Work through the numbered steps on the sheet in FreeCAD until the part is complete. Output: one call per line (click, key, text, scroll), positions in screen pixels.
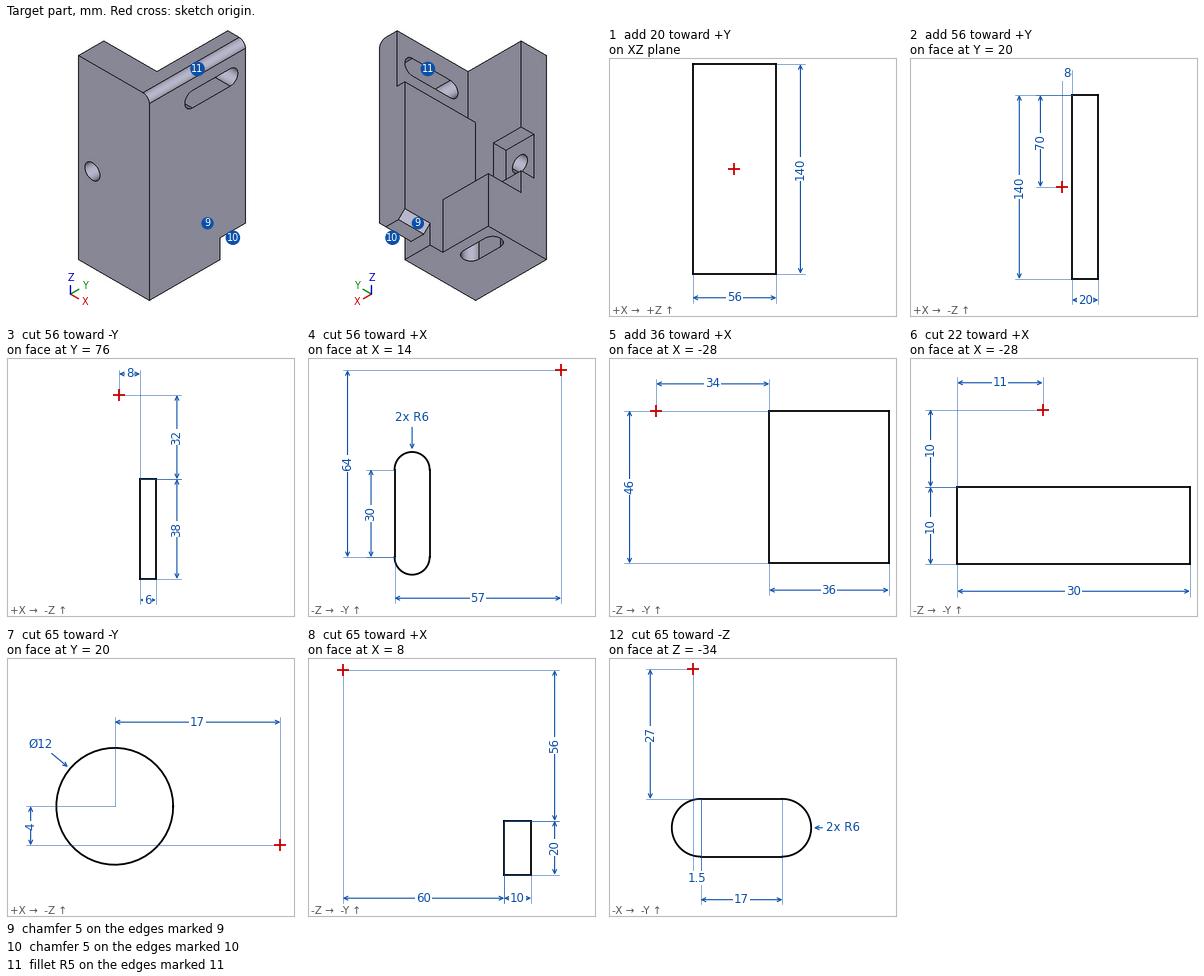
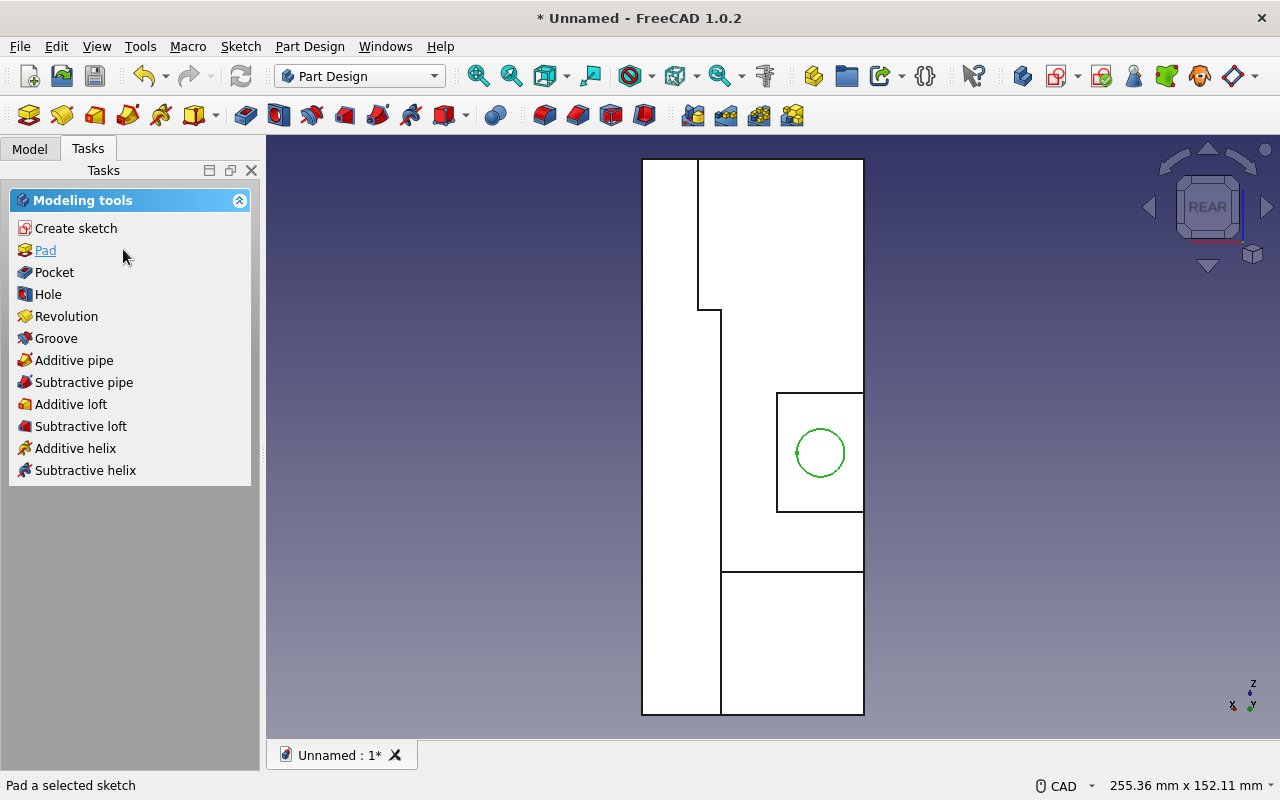
click(246, 116)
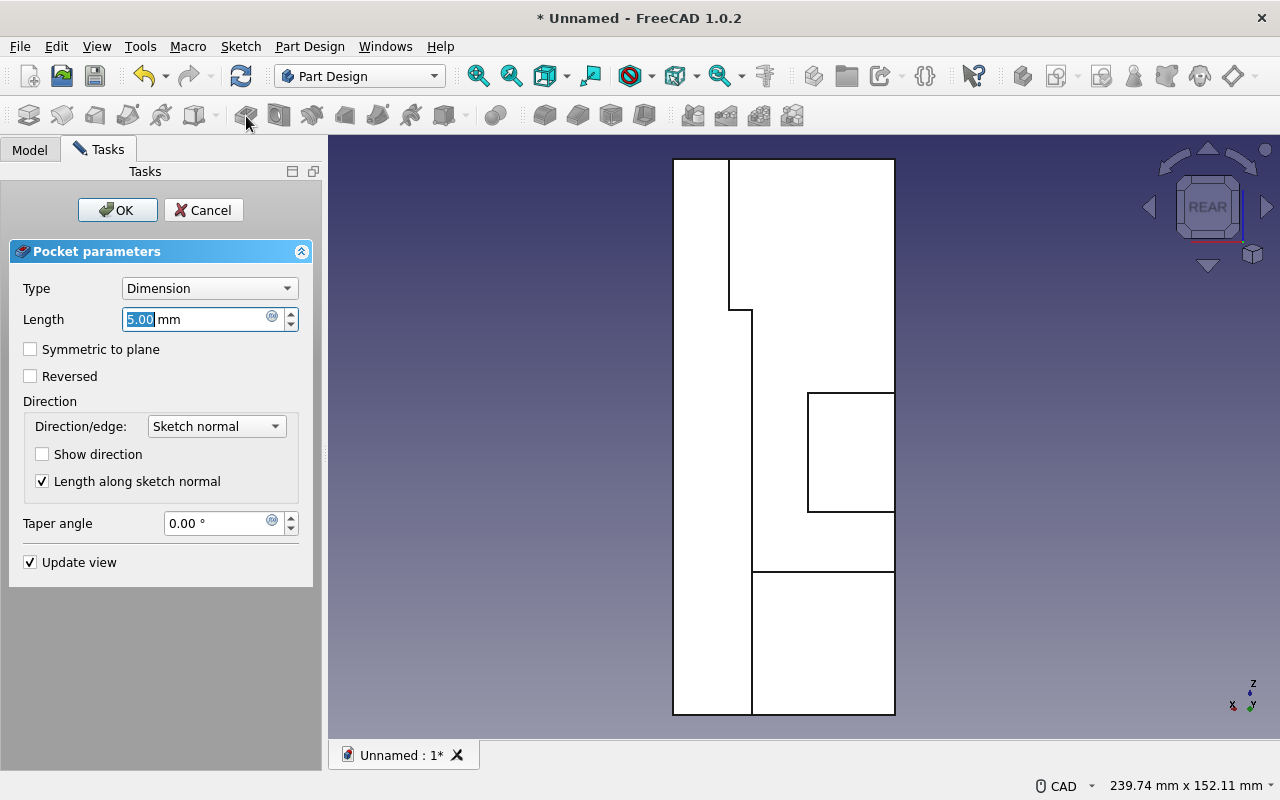
text(65)
key(Tab)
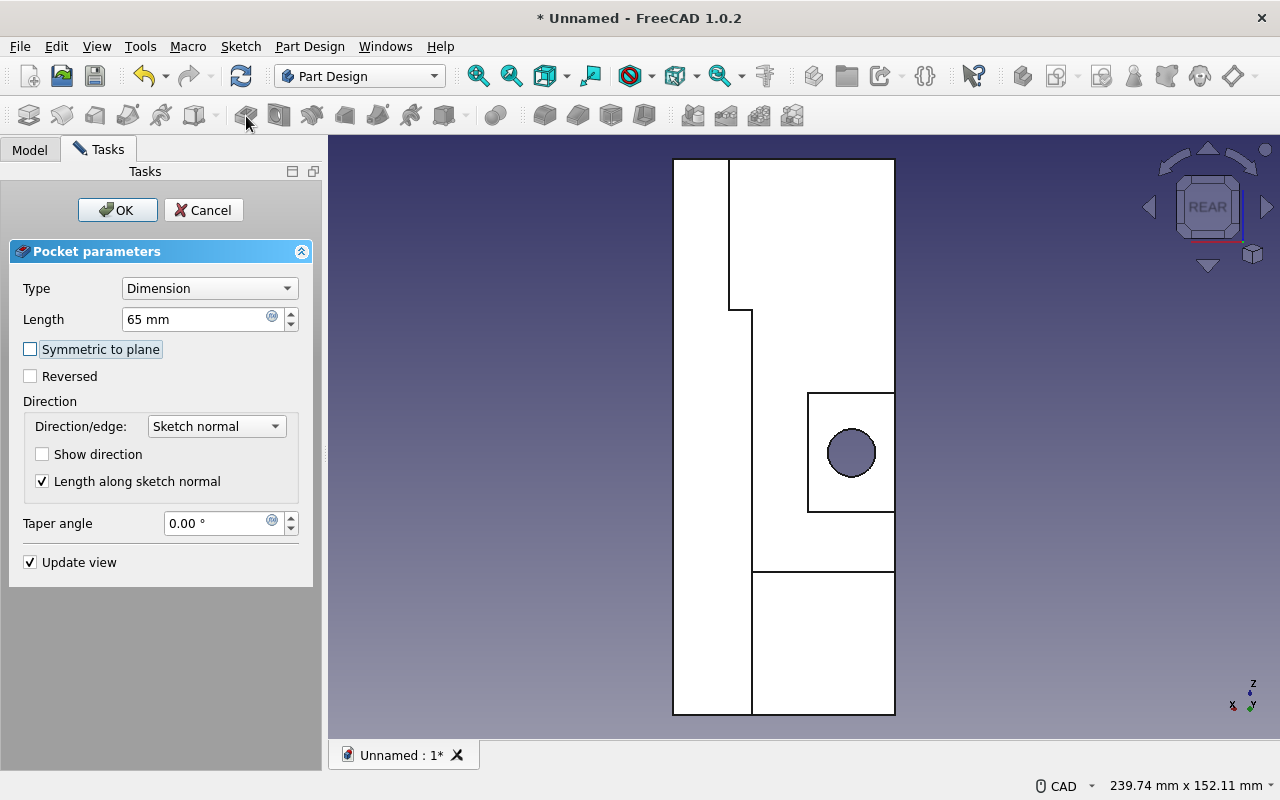
click(118, 210)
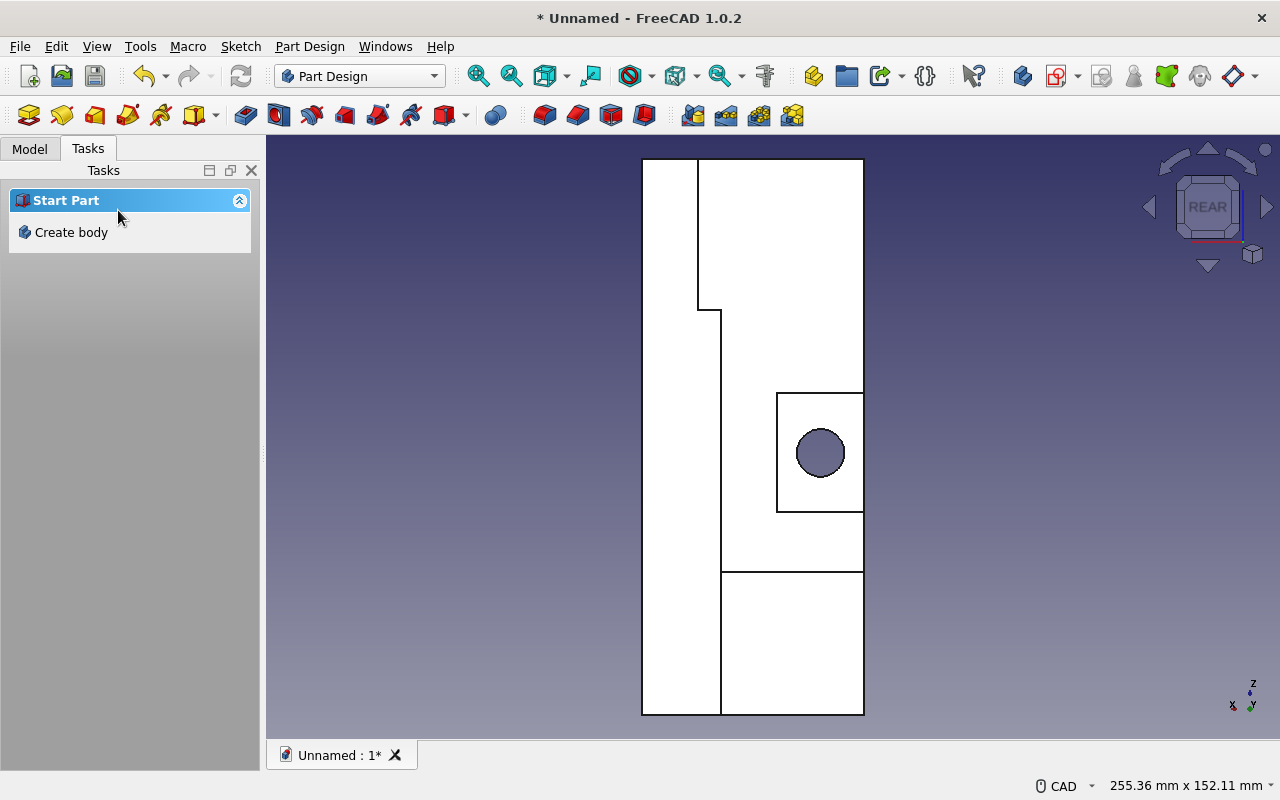
key(6)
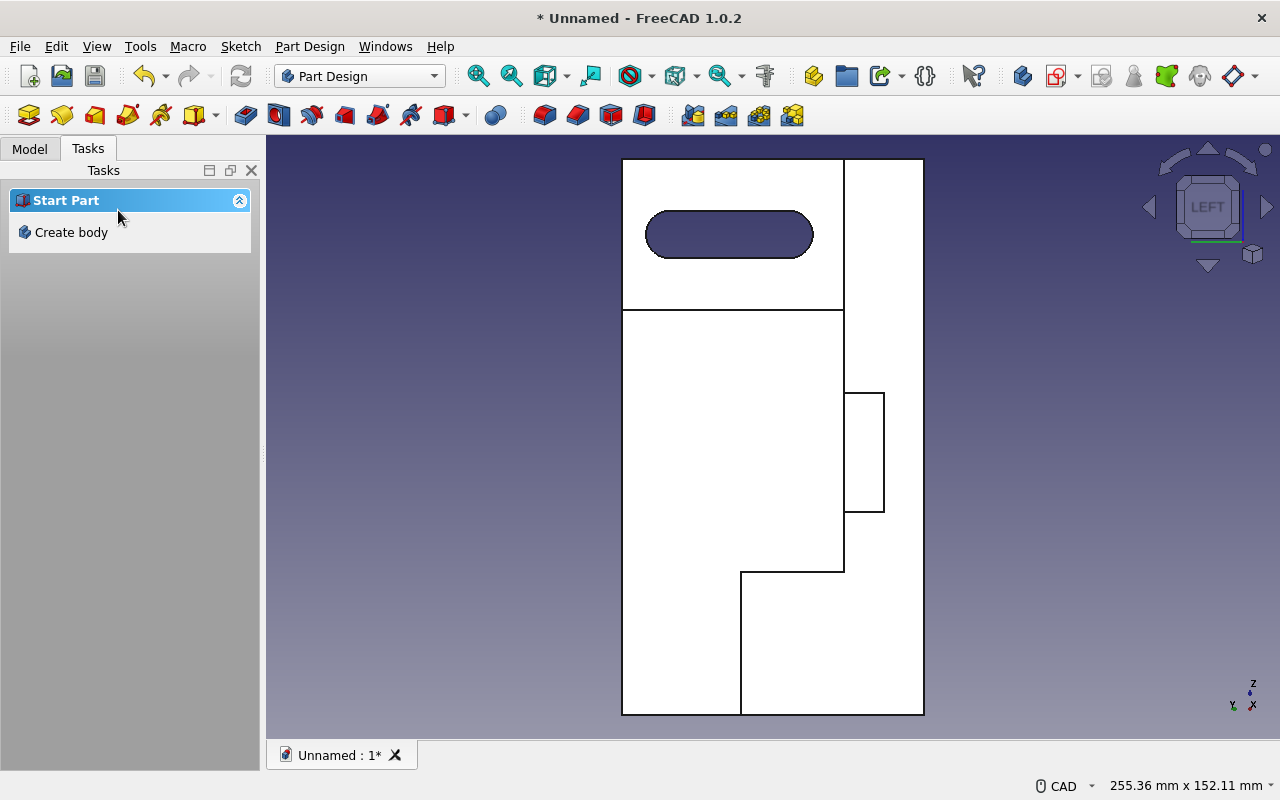
click(733, 454)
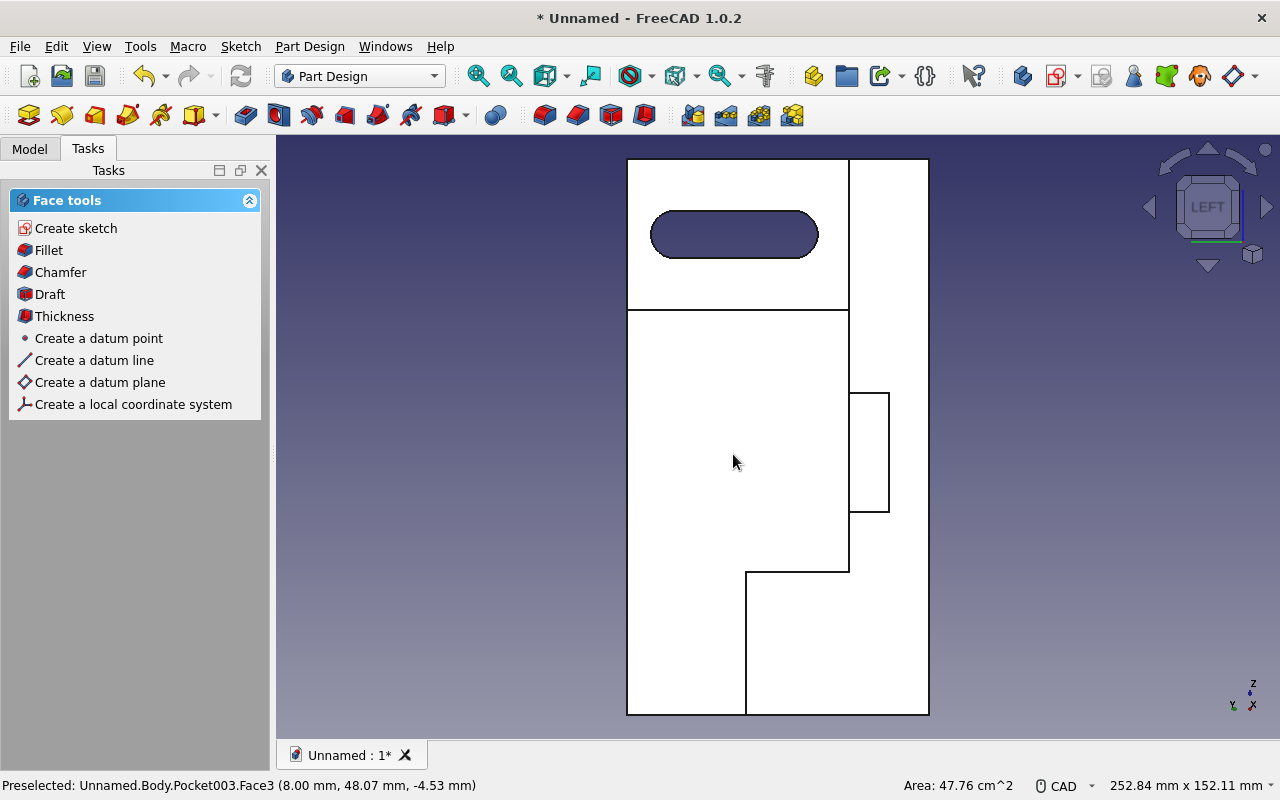
click(1056, 76)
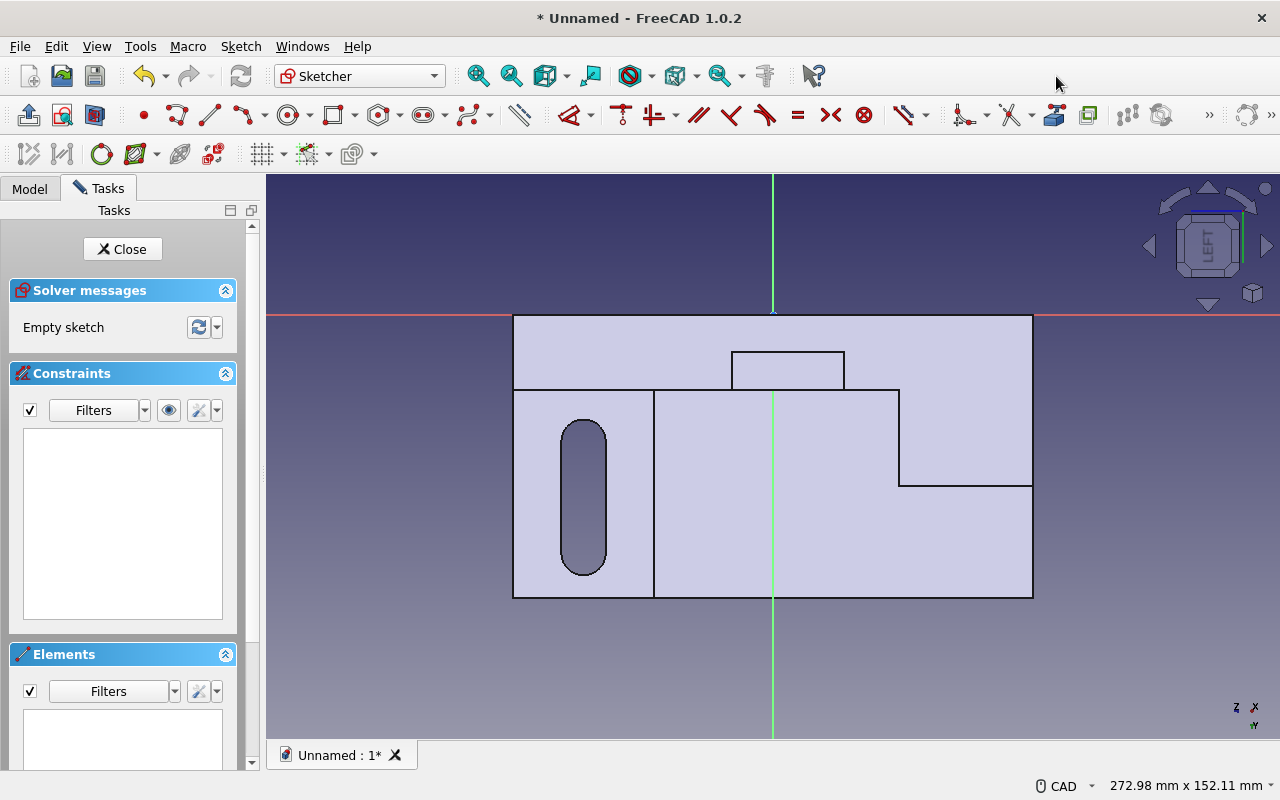
click(95, 116)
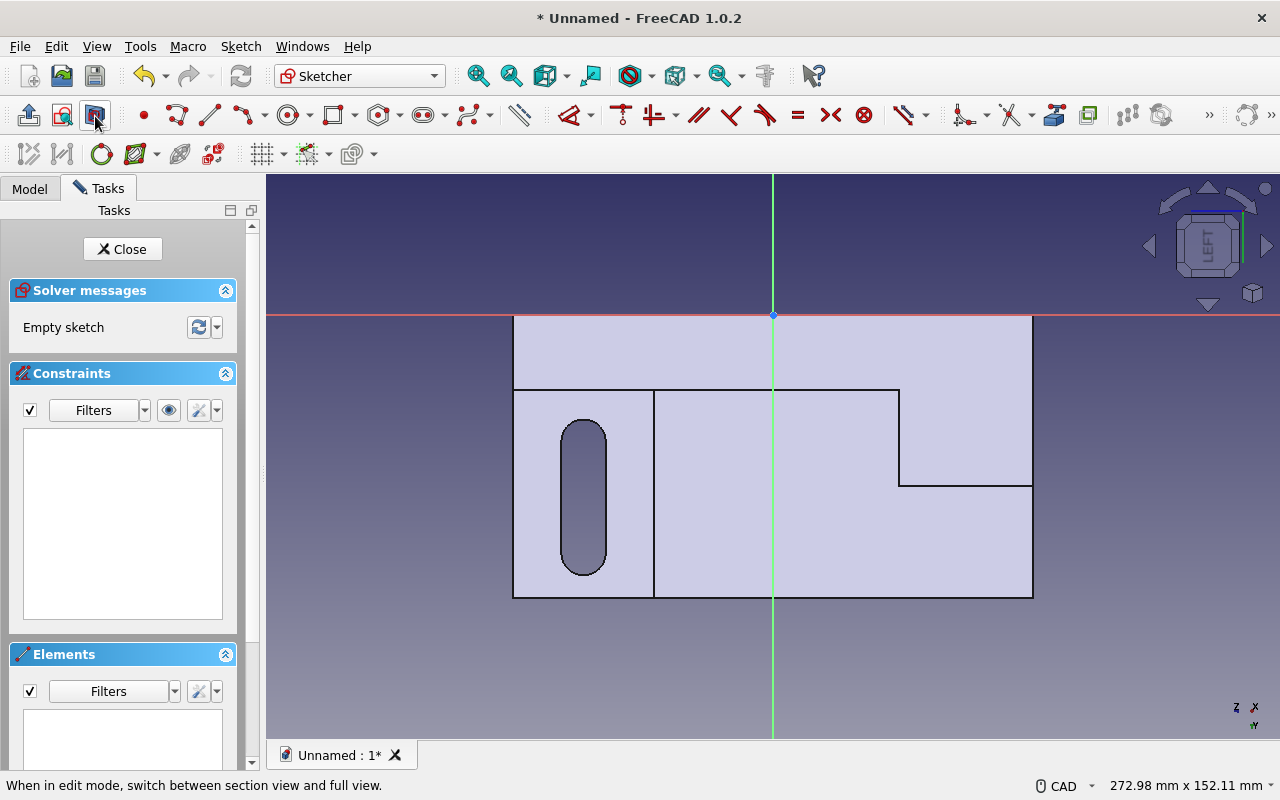
scroll(1093, 587, up, 8)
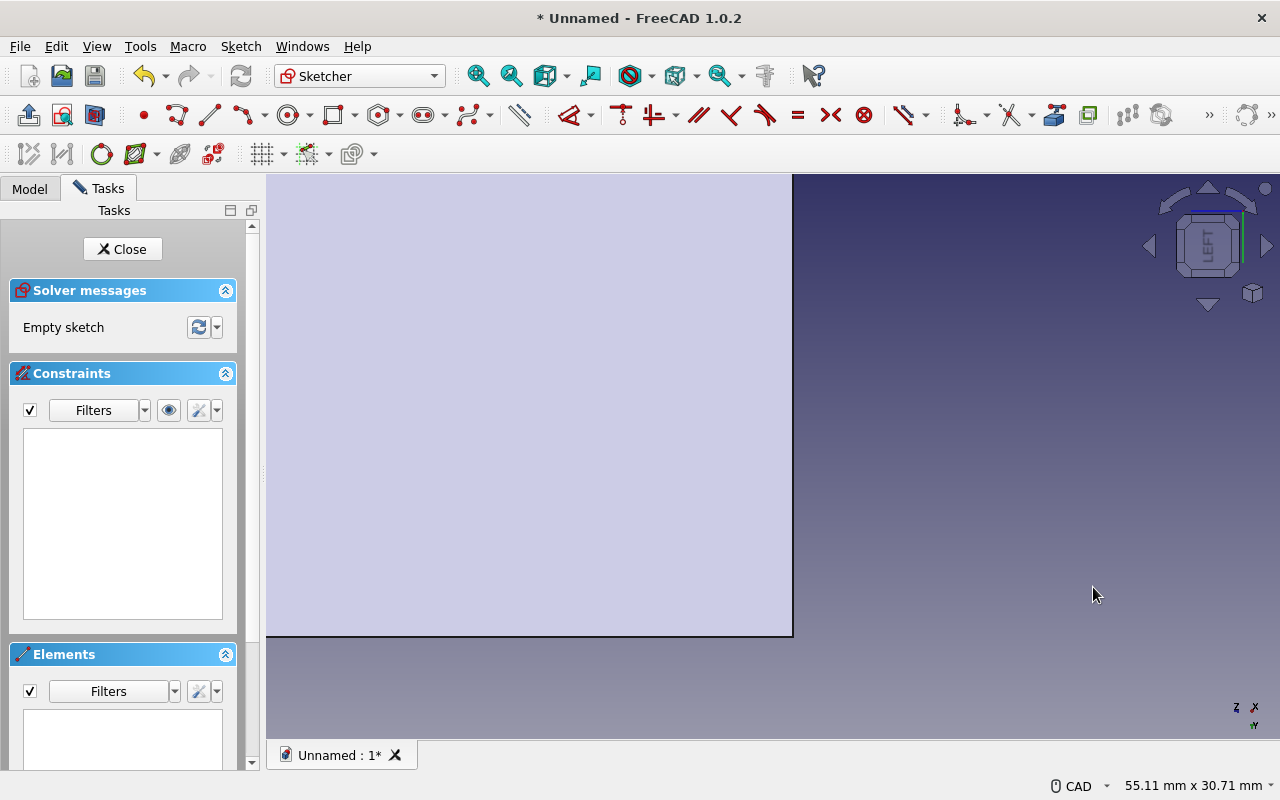
click(332, 116)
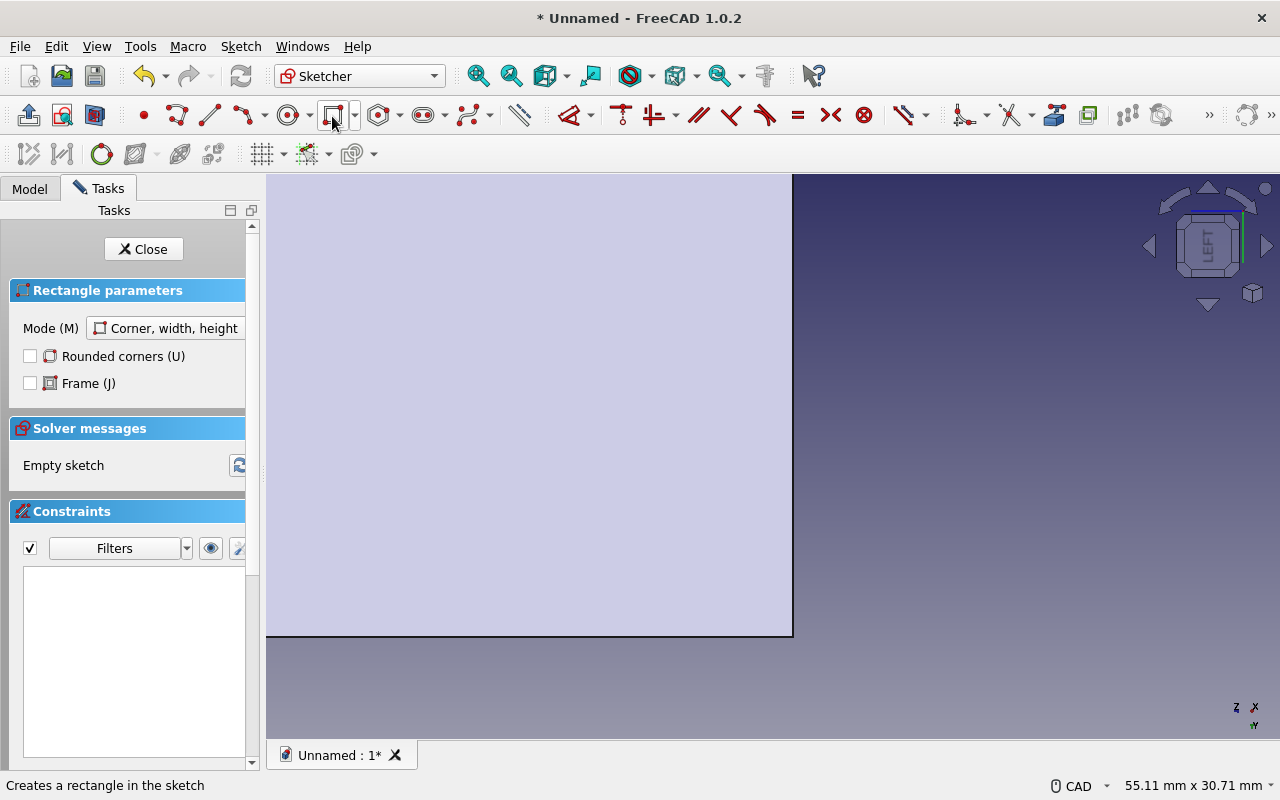
click(609, 269)
click(793, 637)
key(Escape)